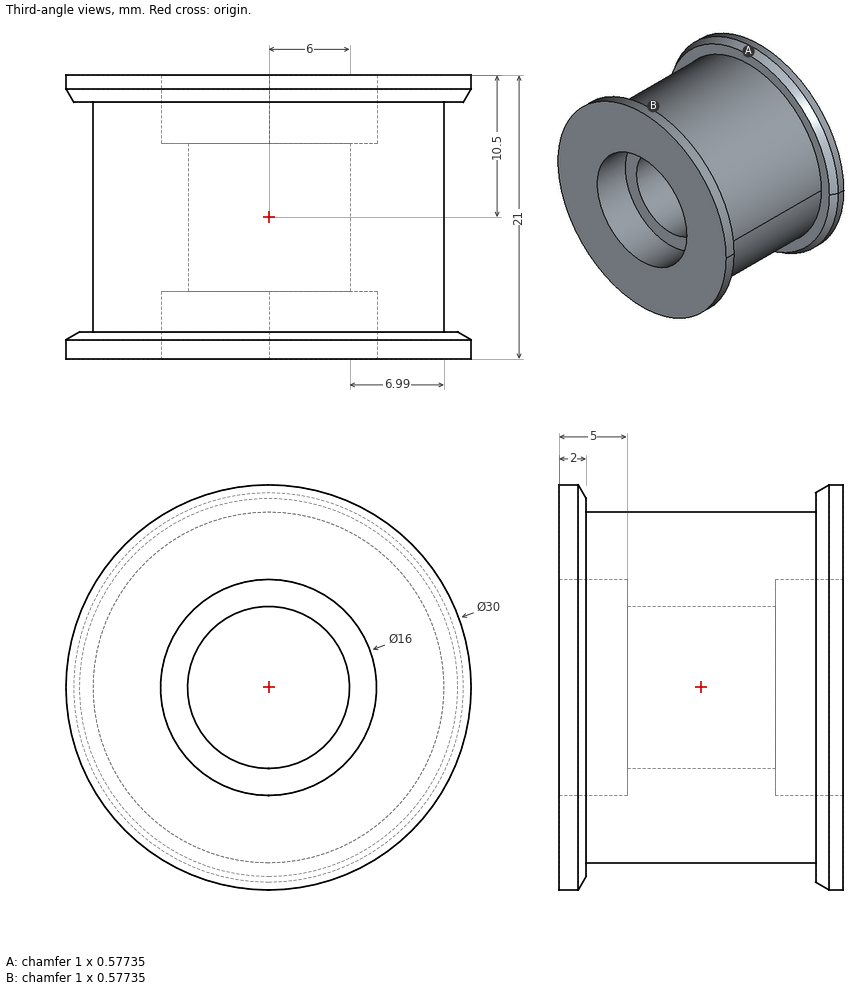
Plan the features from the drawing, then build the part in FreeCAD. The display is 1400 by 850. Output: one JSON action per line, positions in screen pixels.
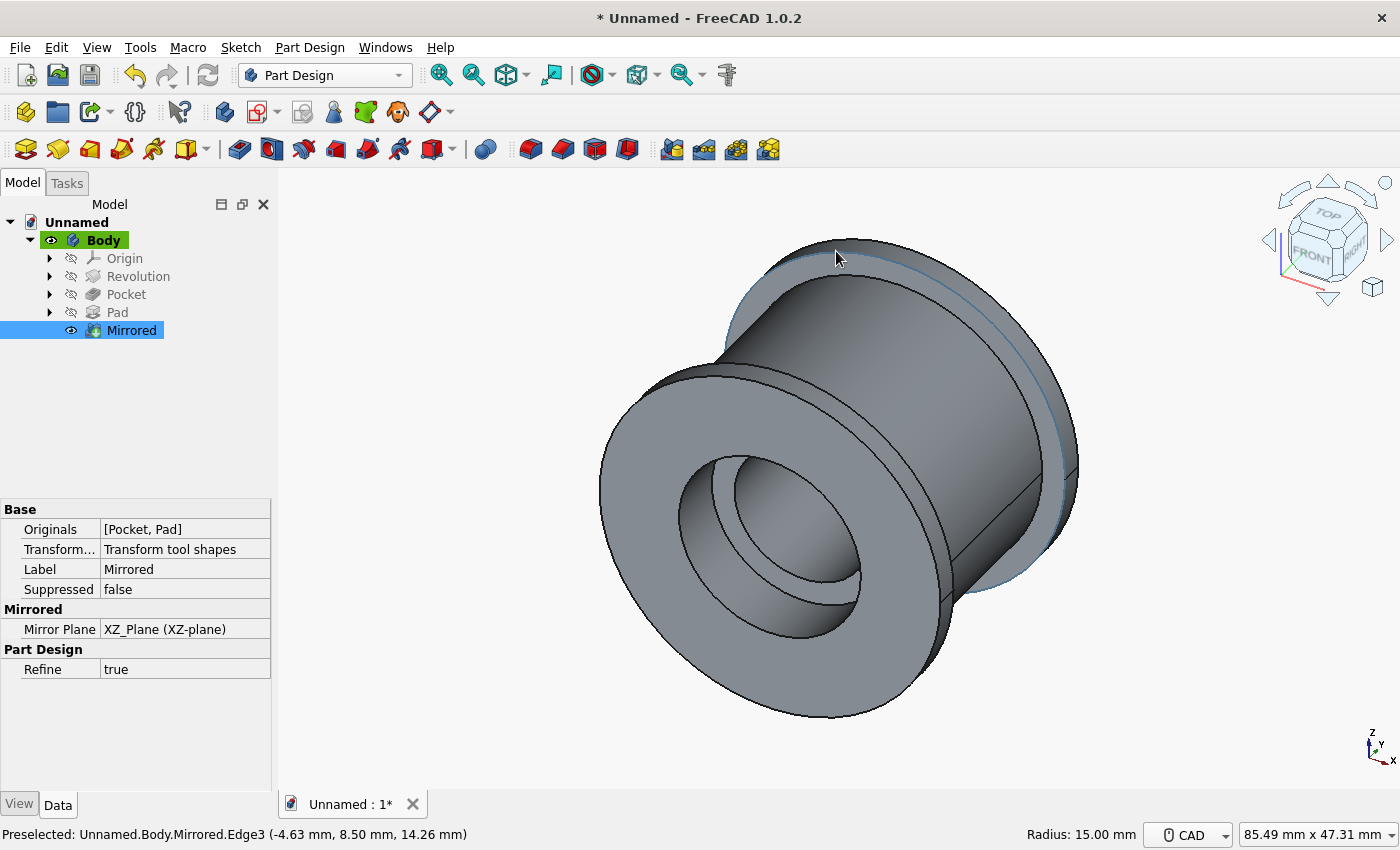
{"action": "left_click", "coordinate": [564, 150]}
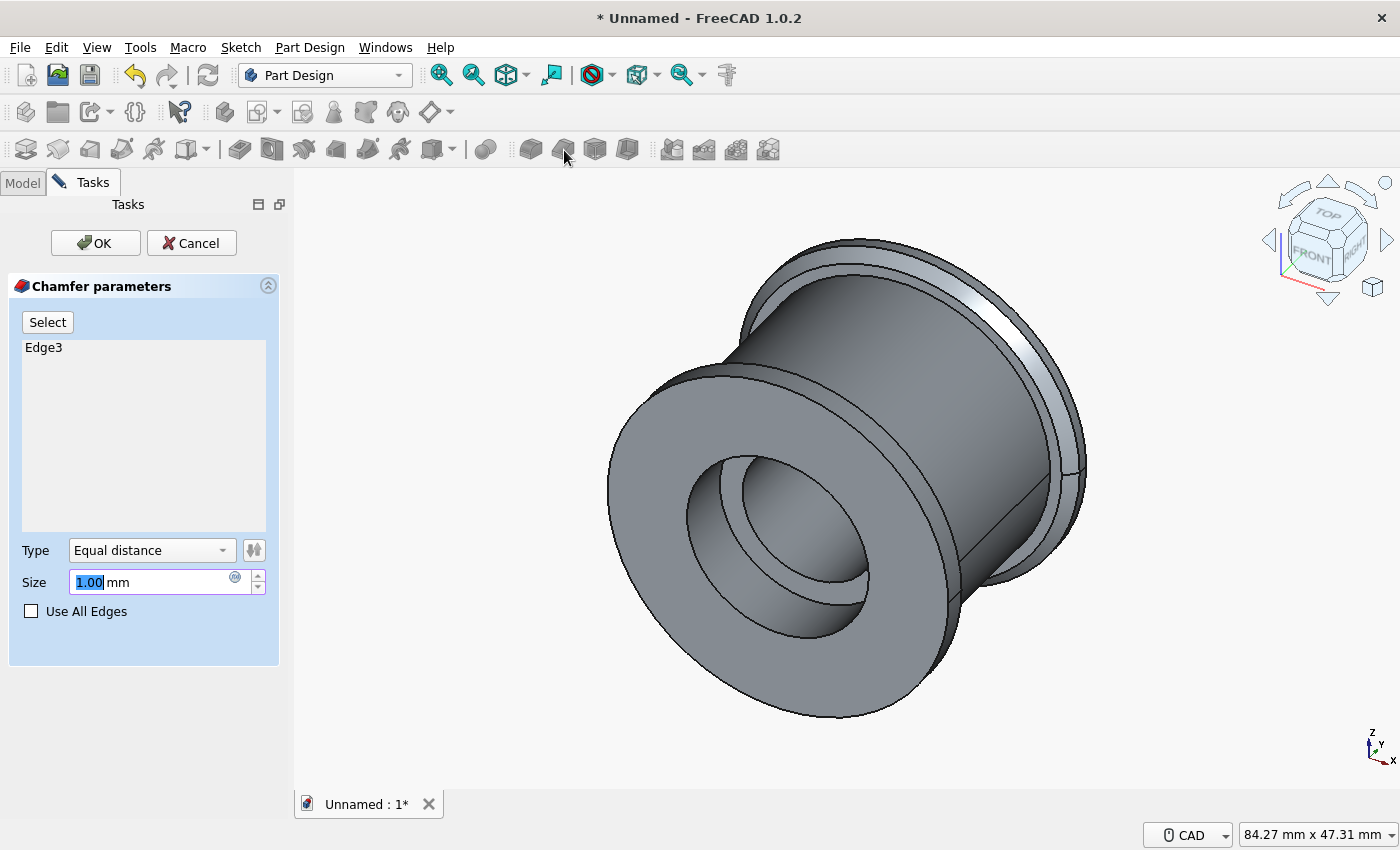
{"action": "type", "text": "1"}
{"action": "key", "text": "Tab"}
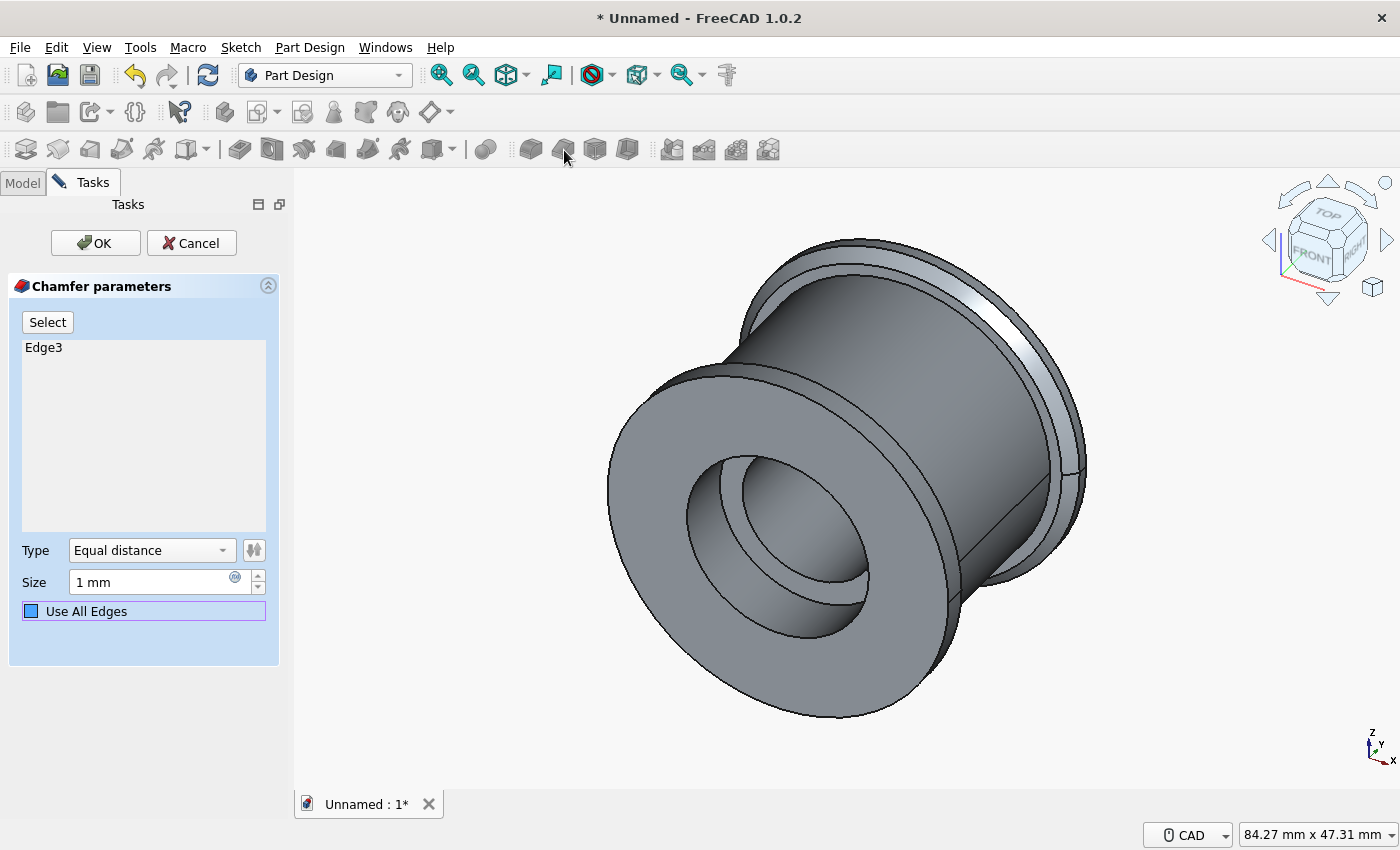
{"action": "left_click", "coordinate": [153, 550]}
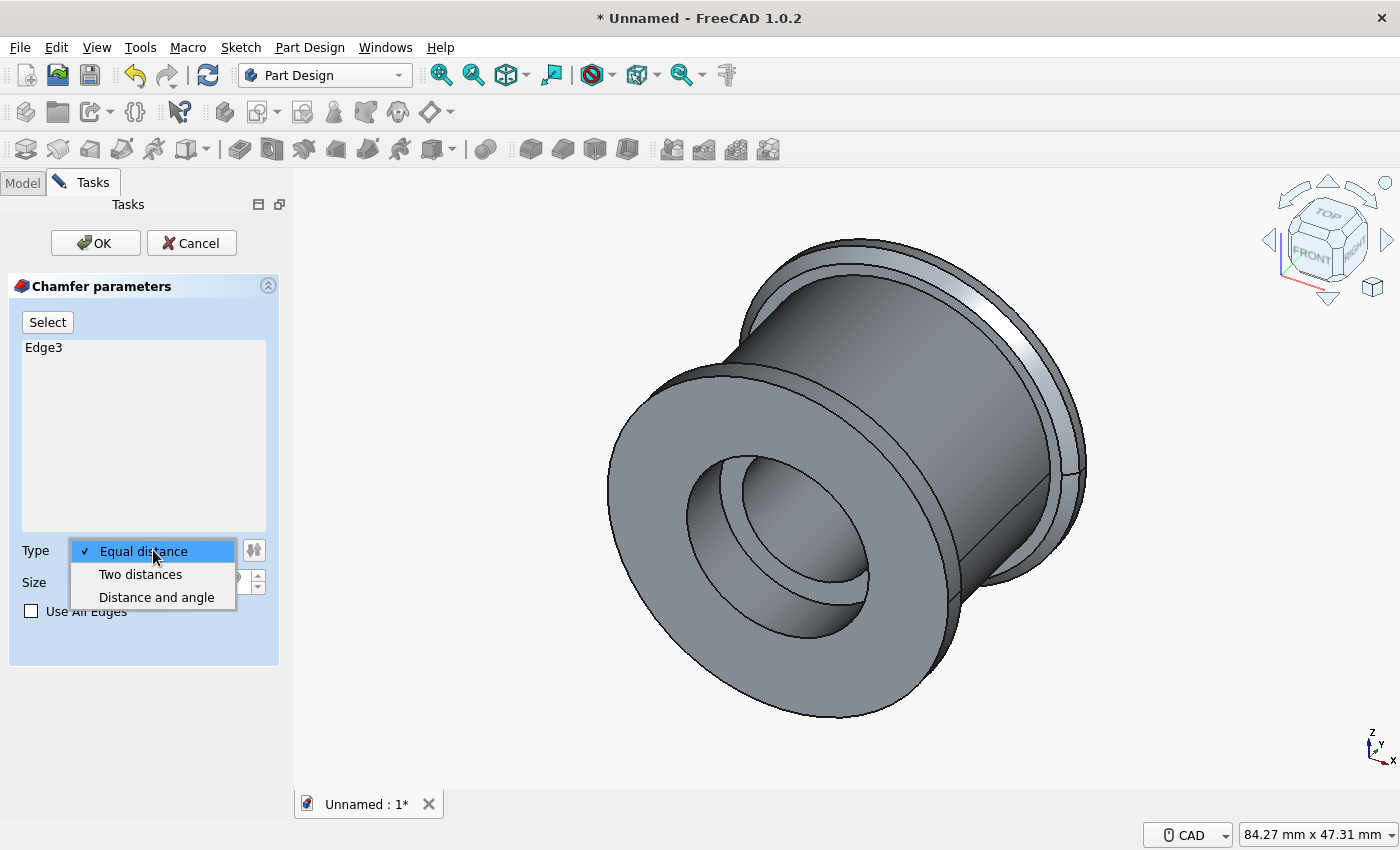
{"action": "left_click", "coordinate": [152, 574]}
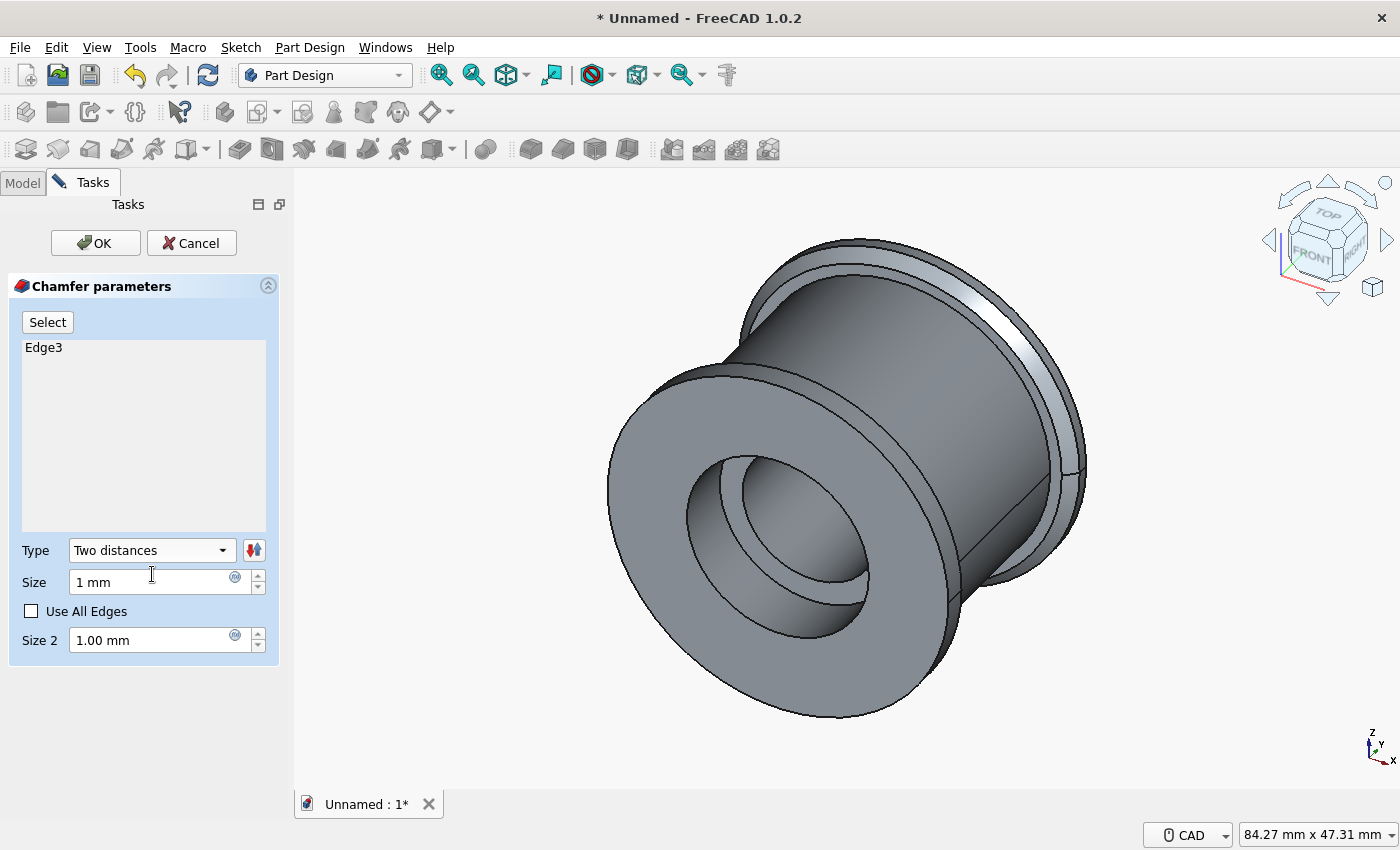
{"action": "triple_click", "coordinate": [160, 640]}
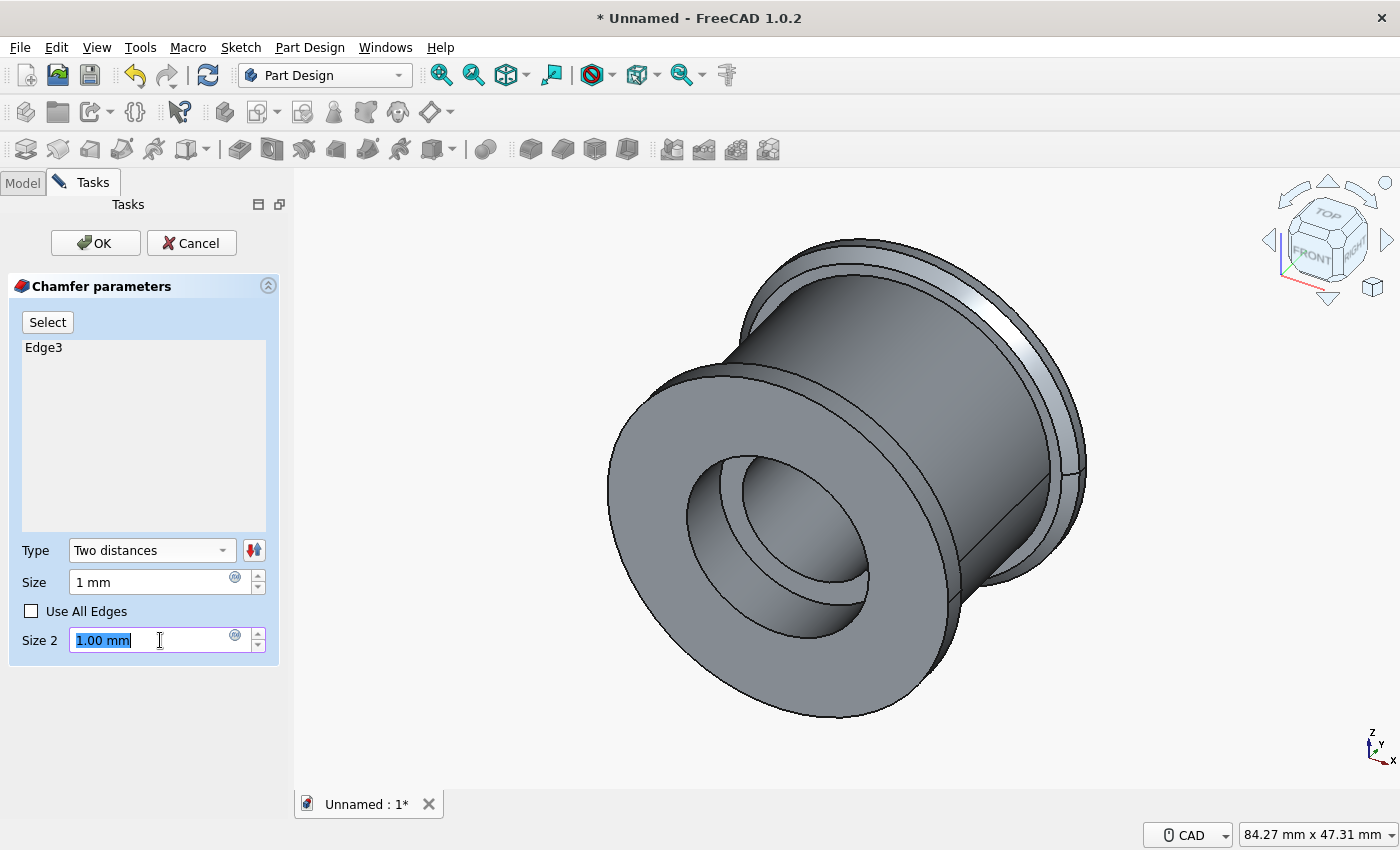
{"action": "type", "text": "0.57735"}
{"action": "key", "text": "Tab"}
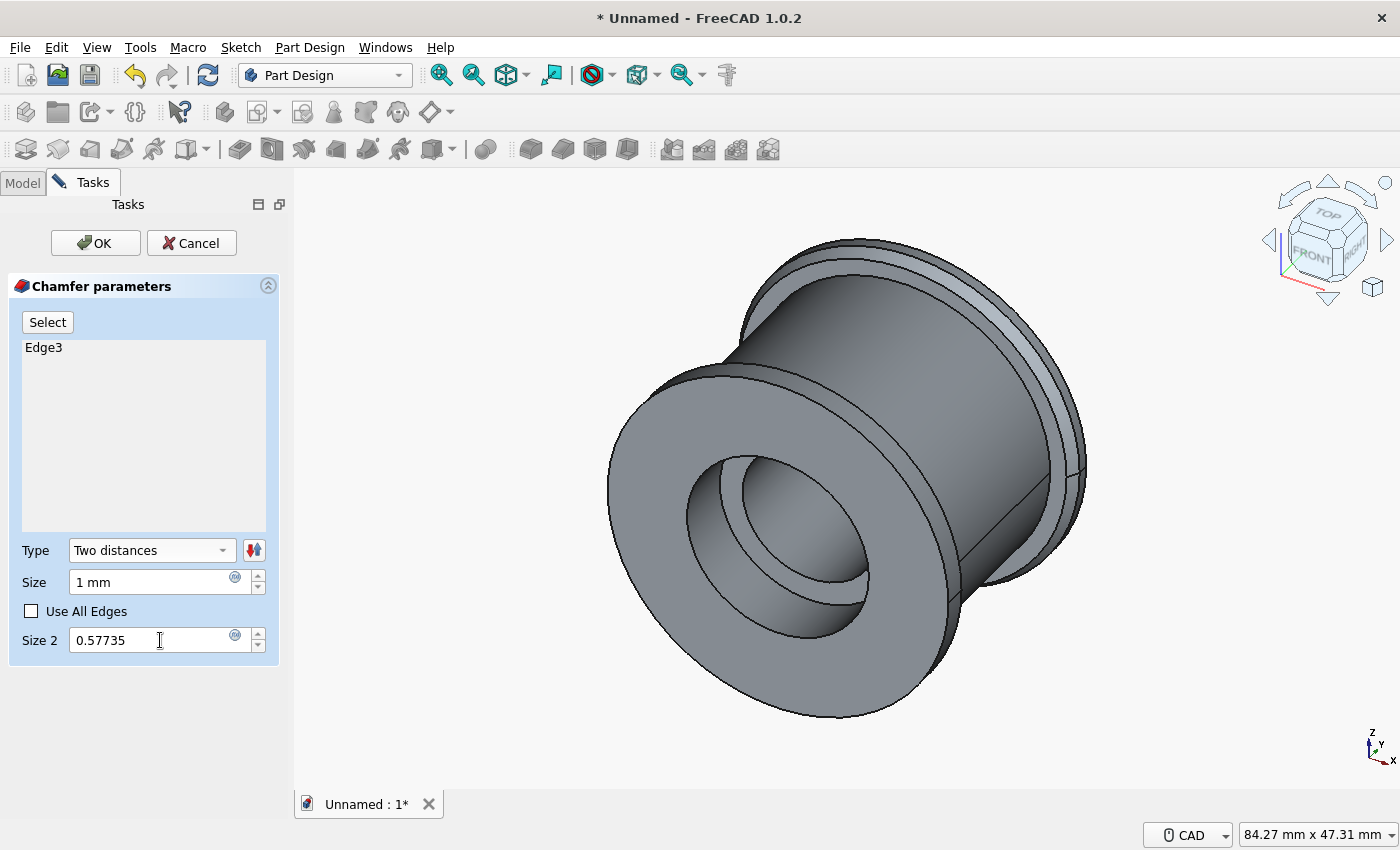
{"action": "left_click", "coordinate": [96, 243]}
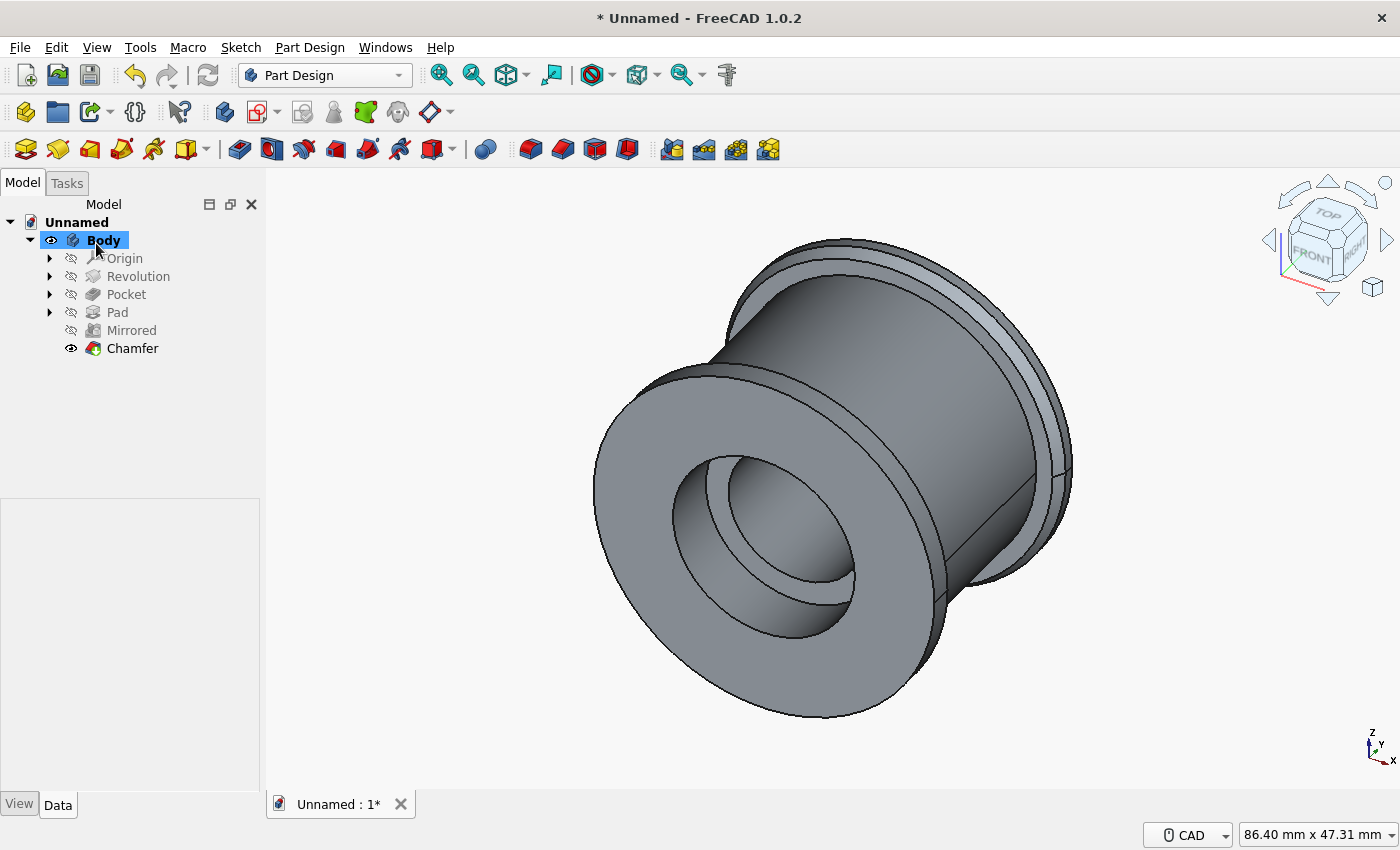
{"action": "key", "text": "0"}